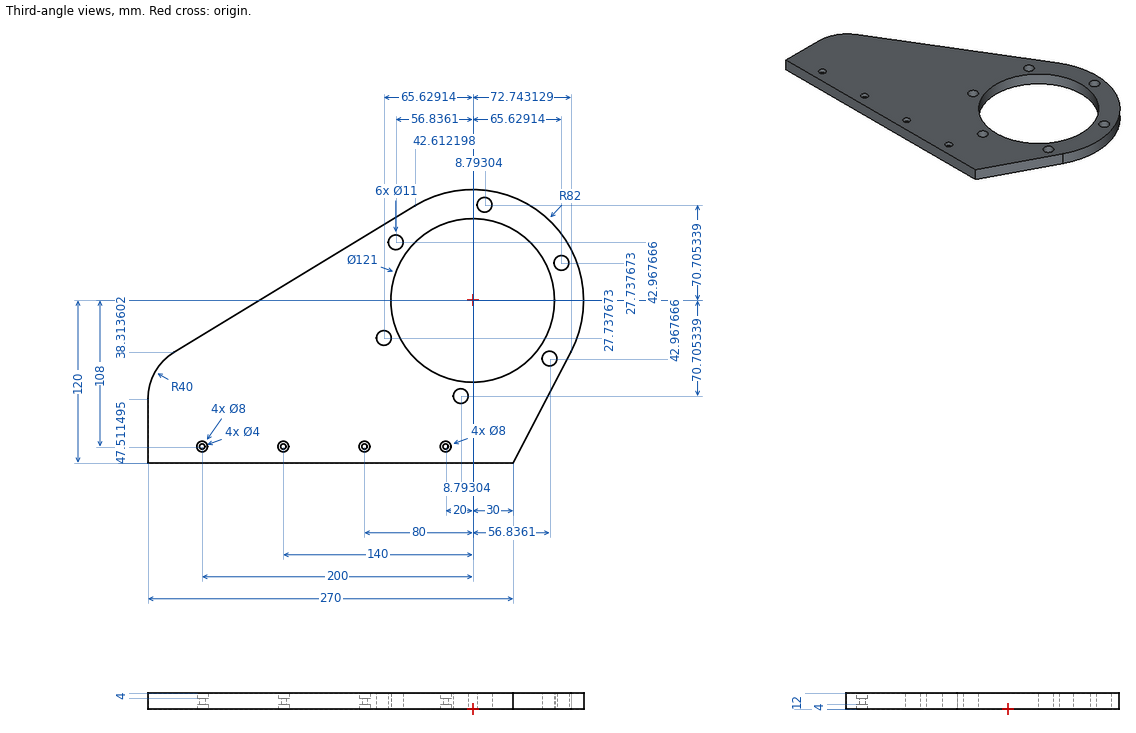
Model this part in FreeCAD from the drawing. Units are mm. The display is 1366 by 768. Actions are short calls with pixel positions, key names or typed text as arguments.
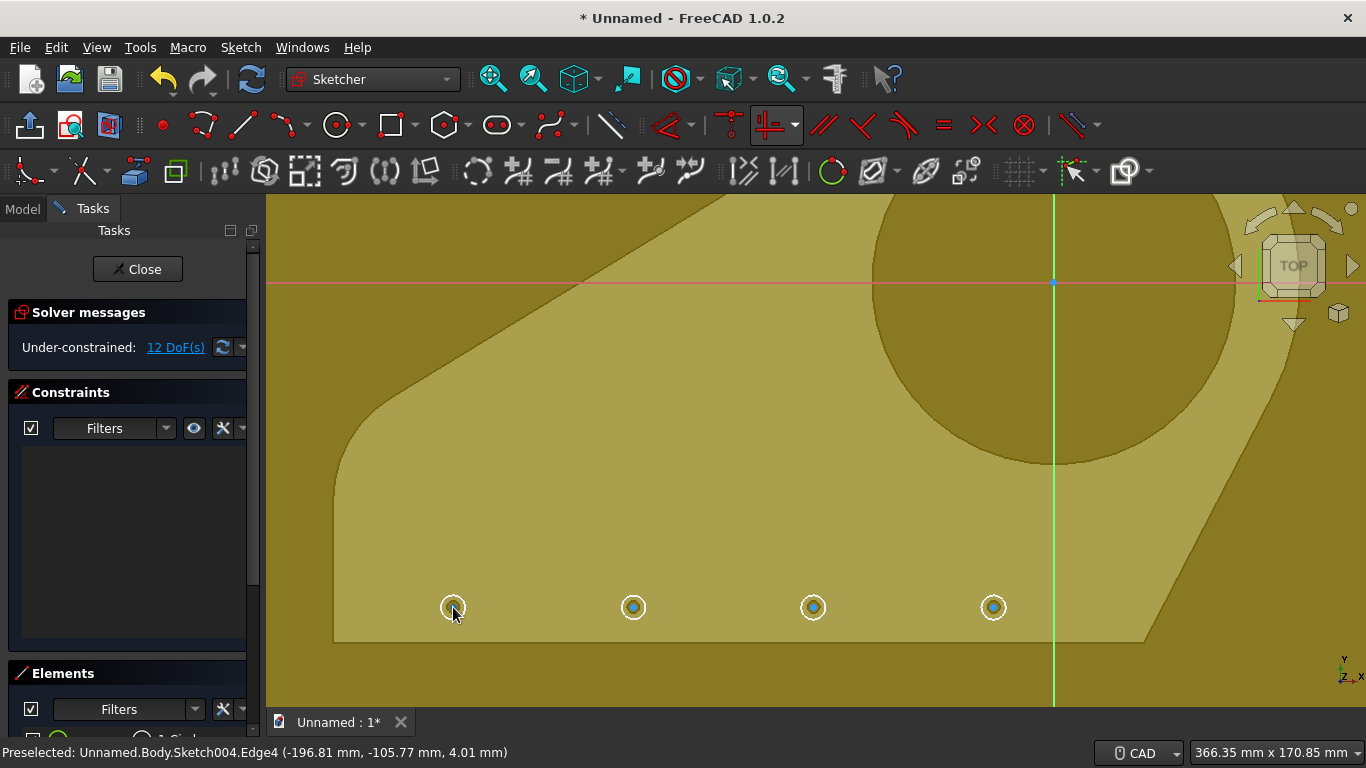
click(1002, 599)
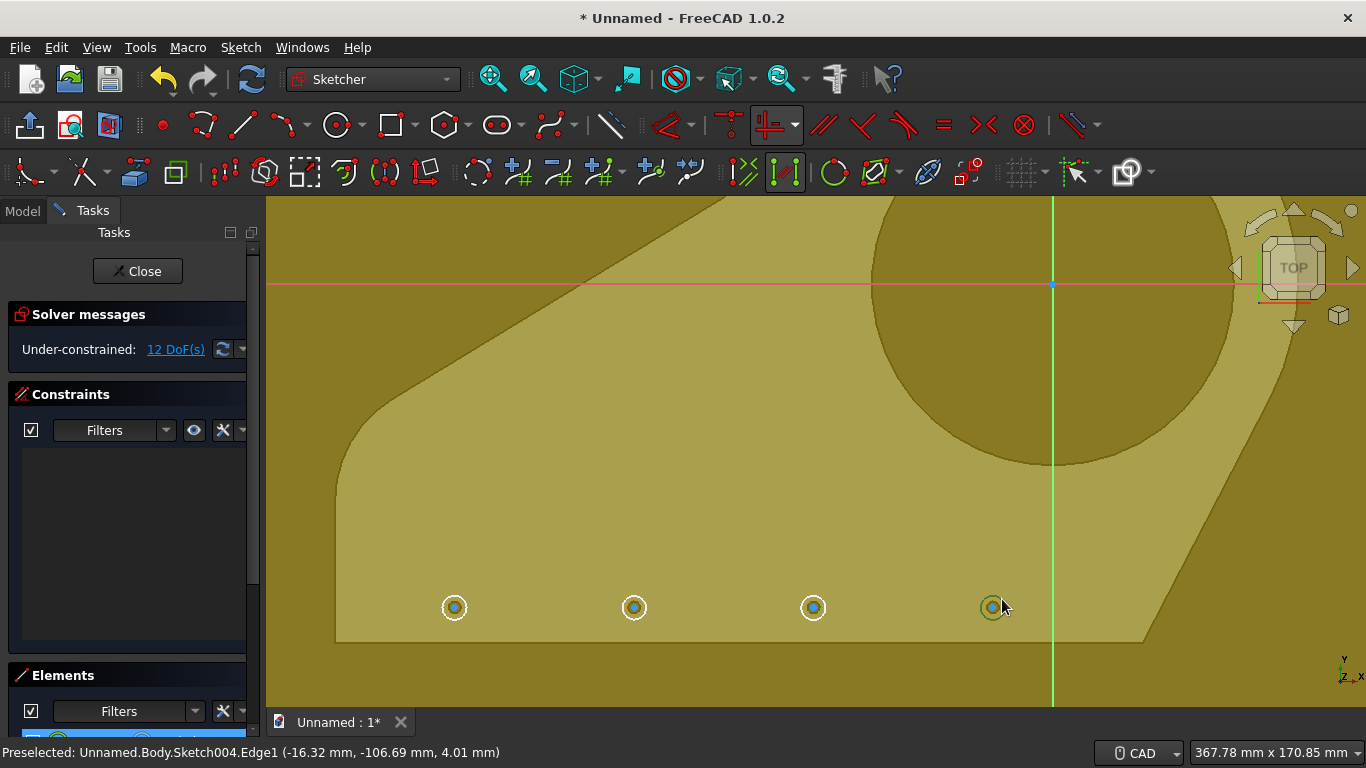
click(822, 599)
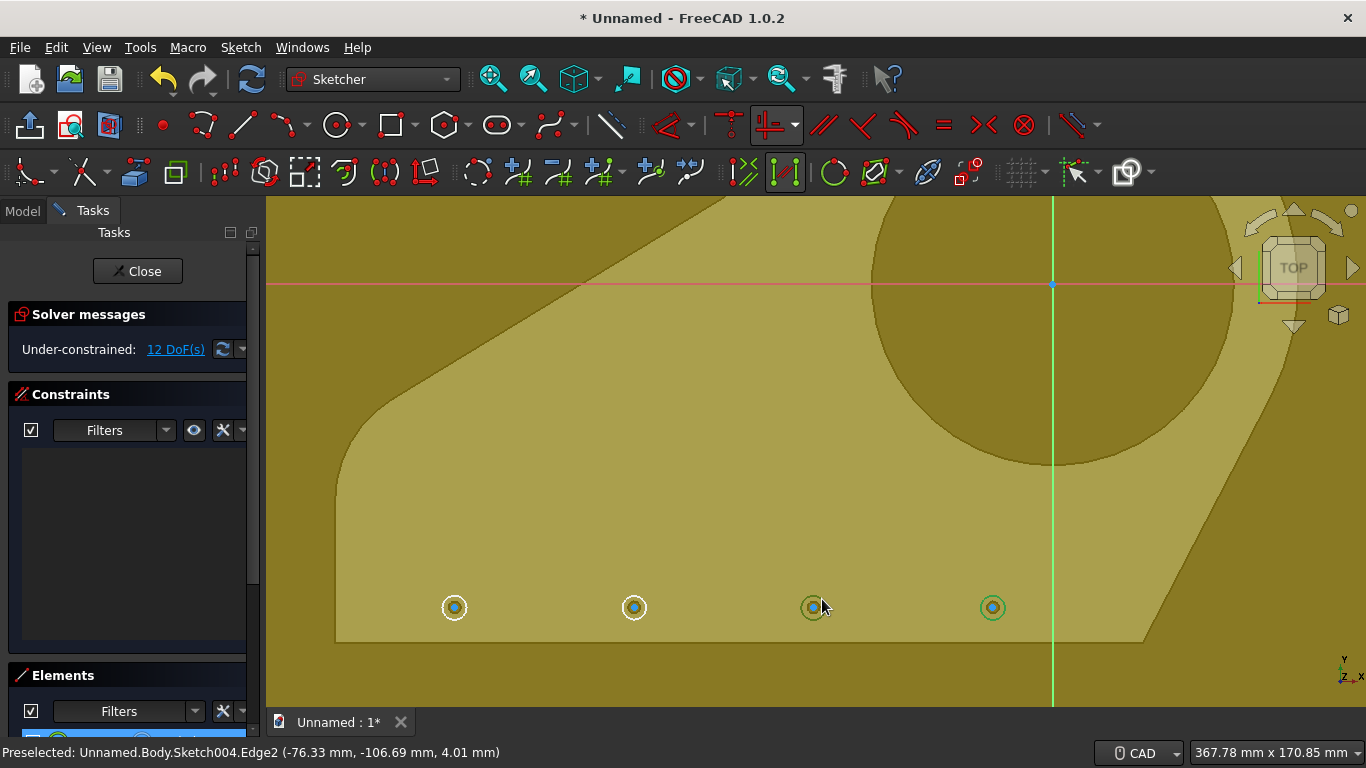
click(643, 600)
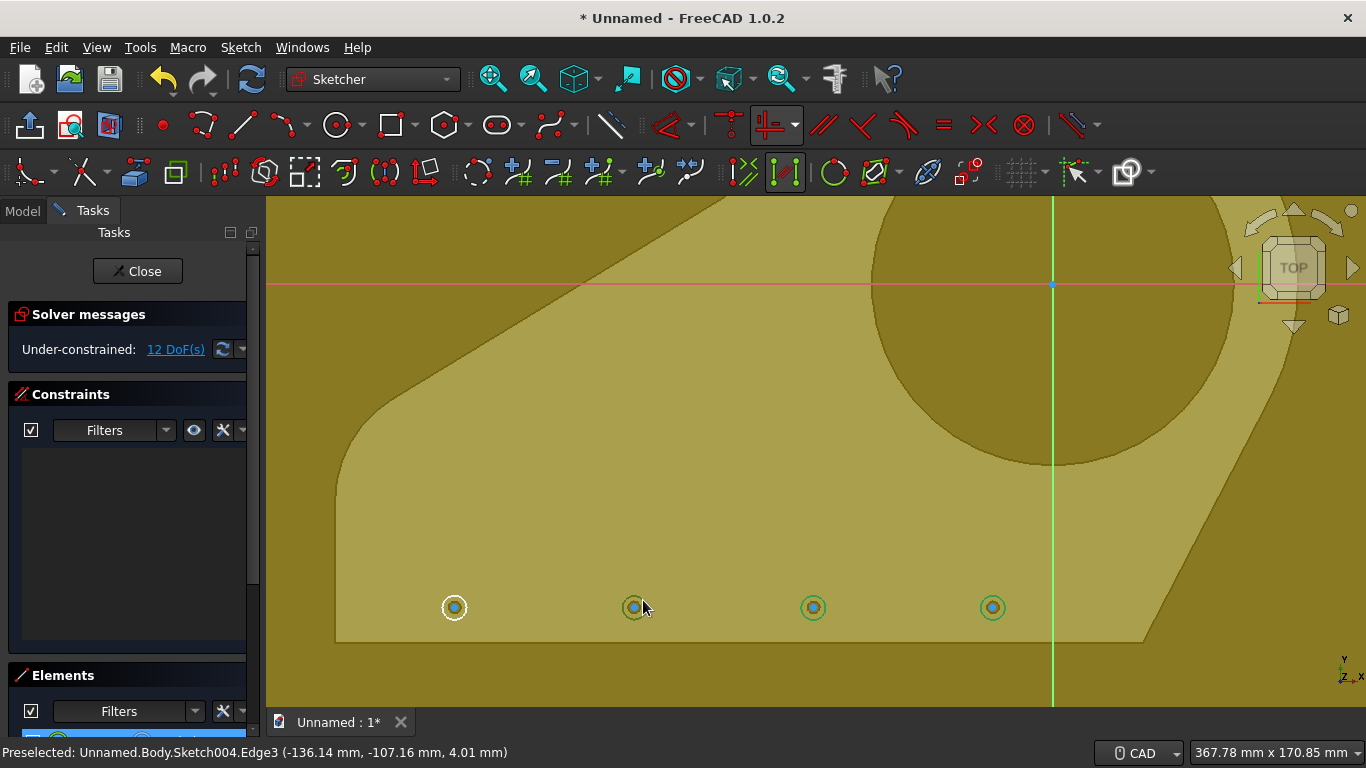
click(463, 599)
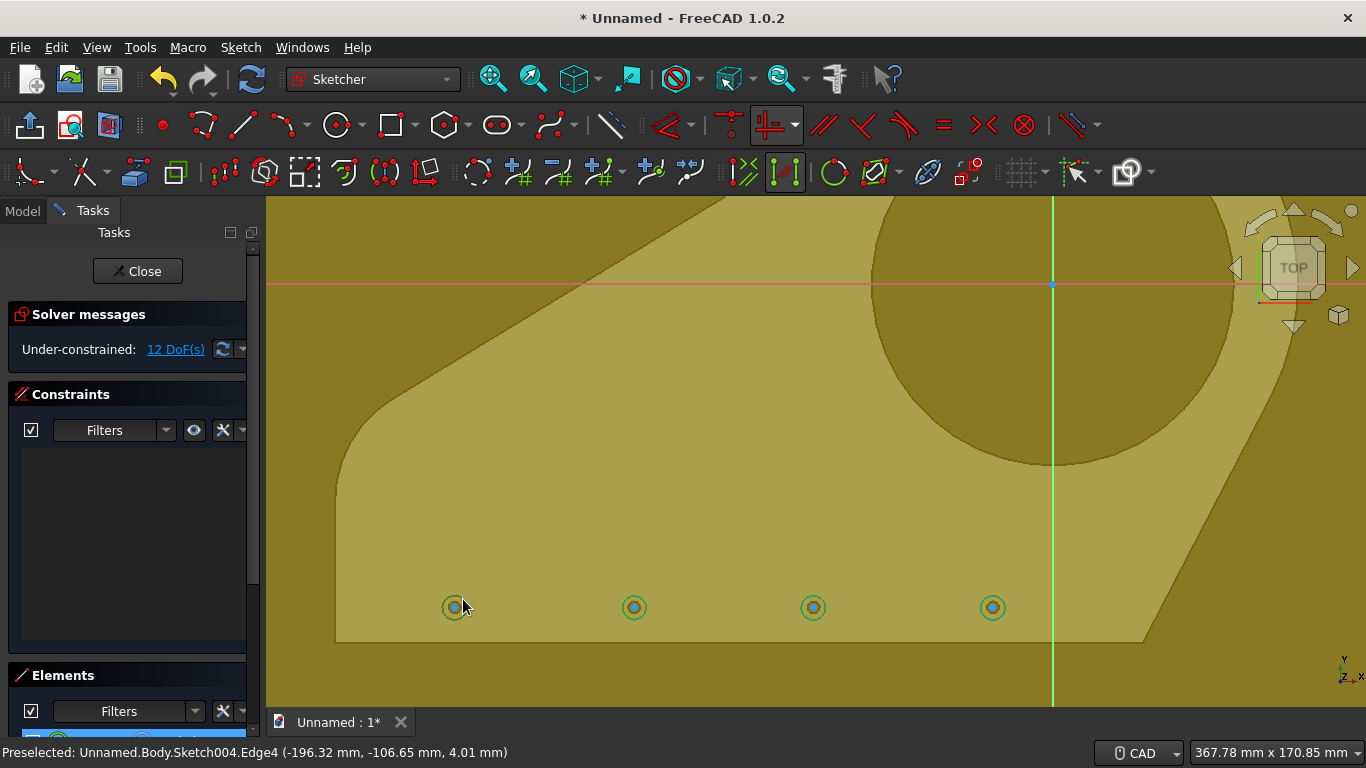
click(944, 126)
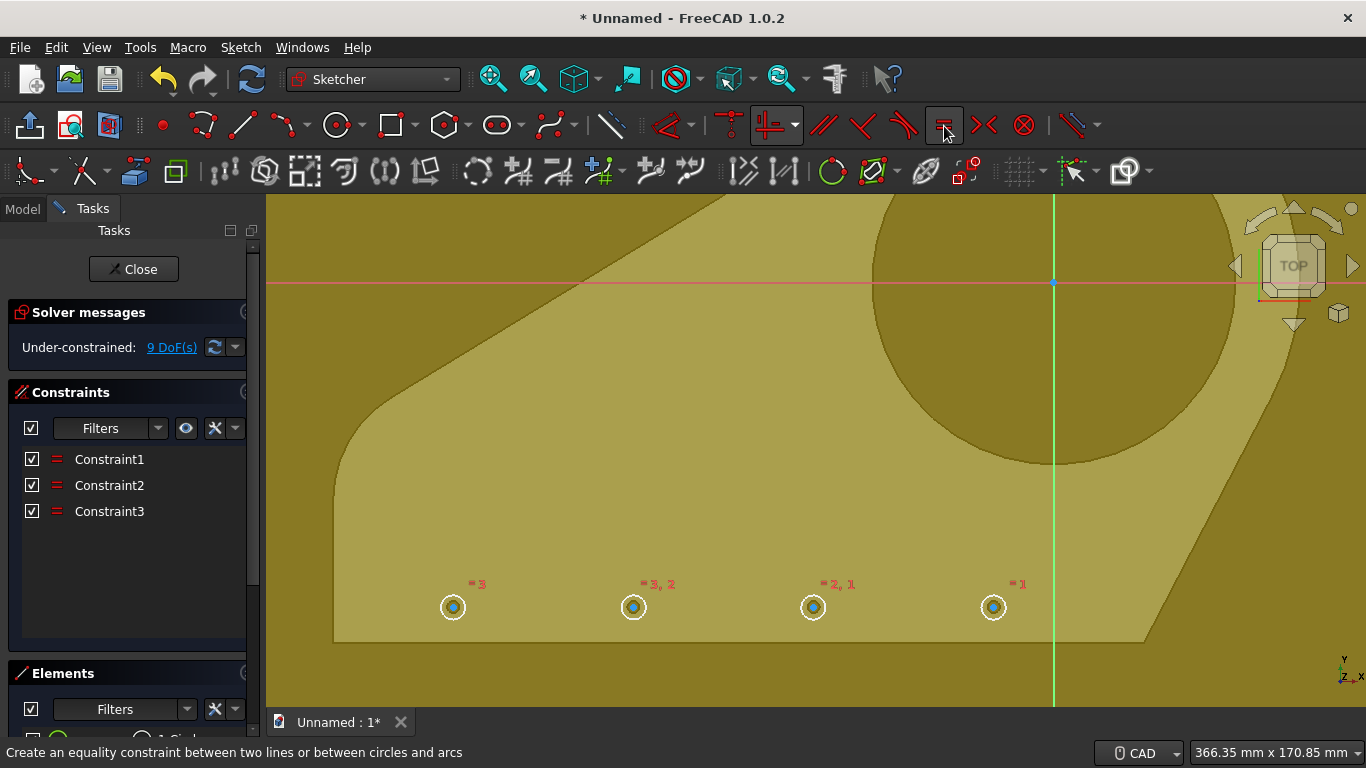
click(994, 608)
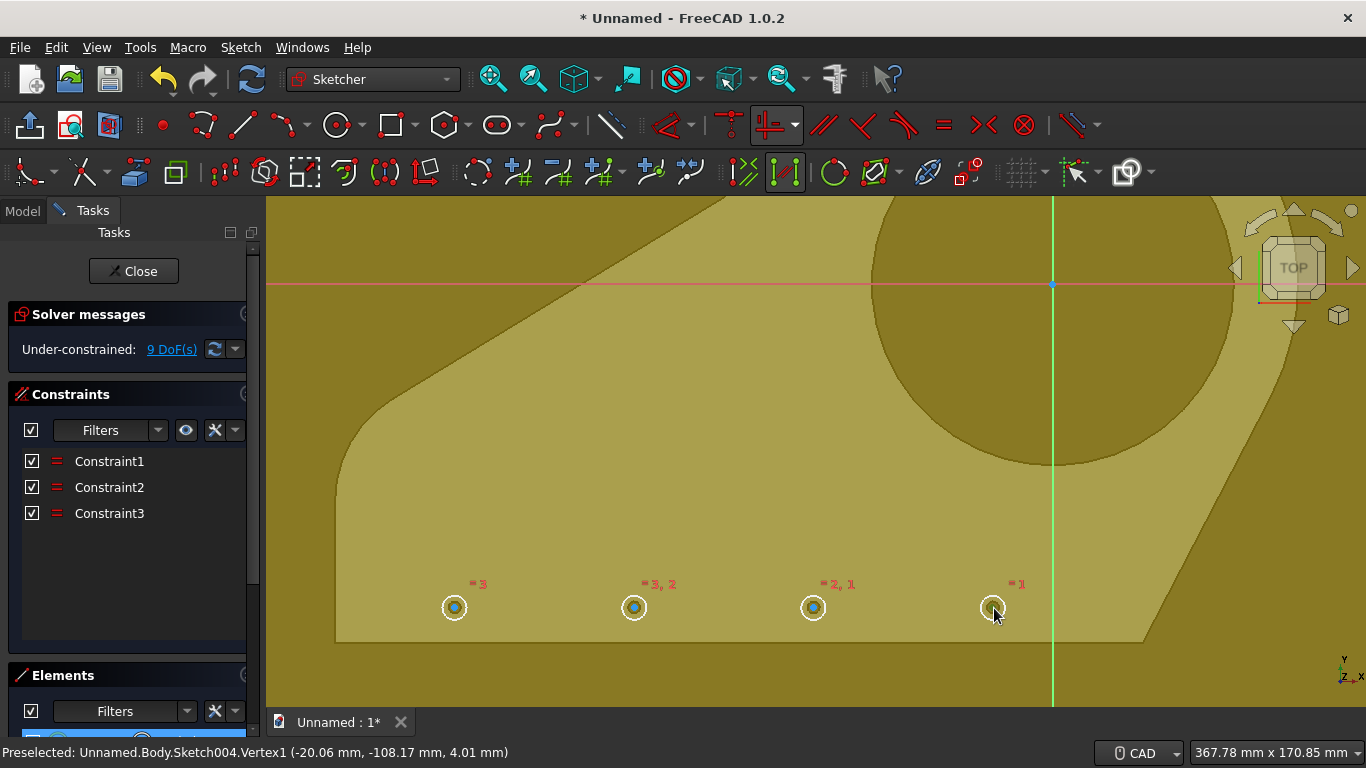
click(813, 608)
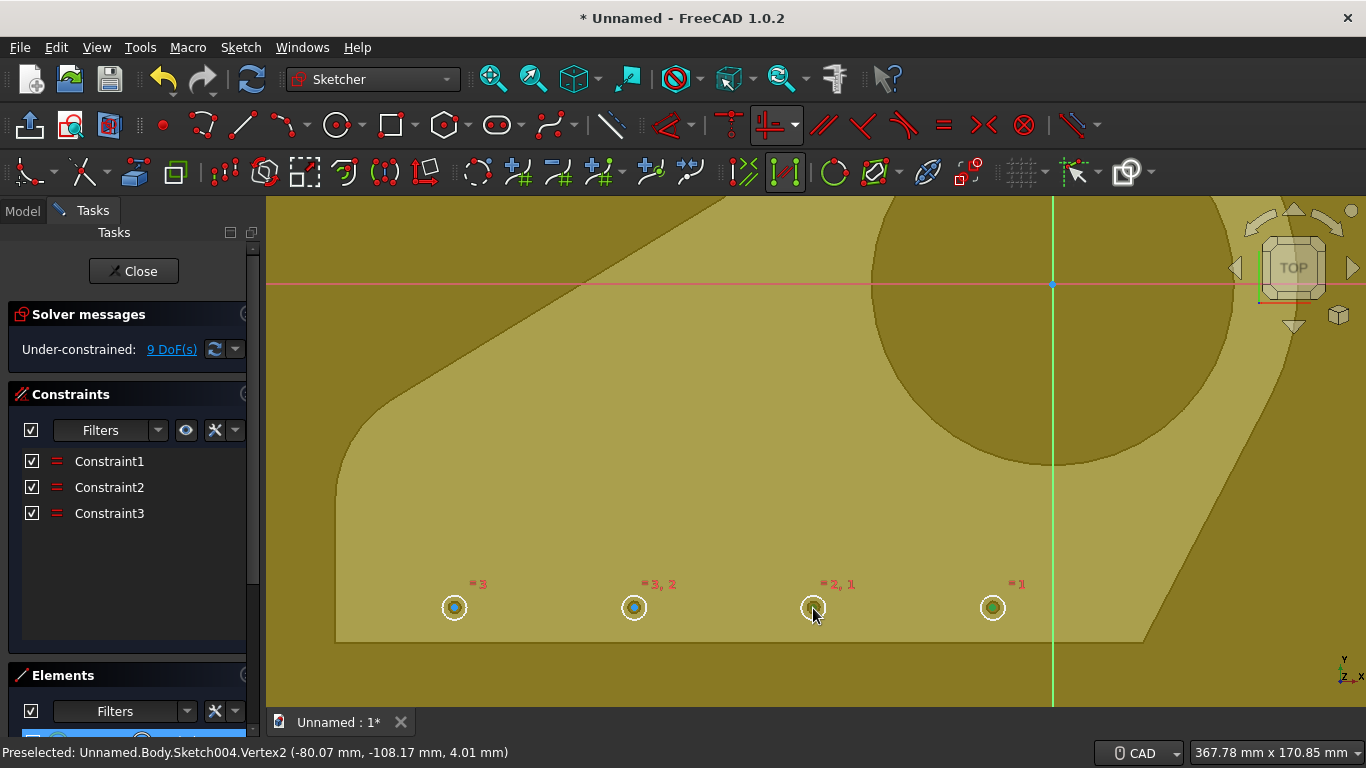
key(h)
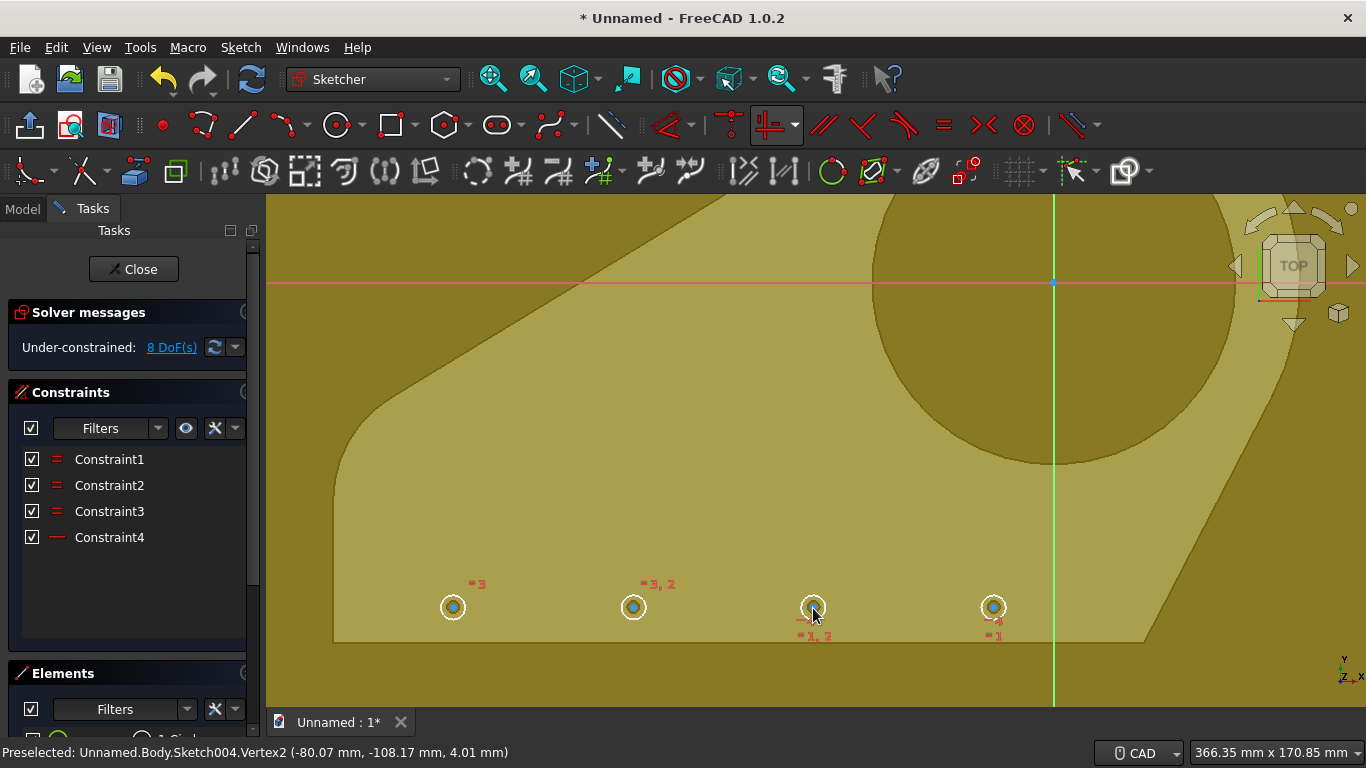
click(813, 608)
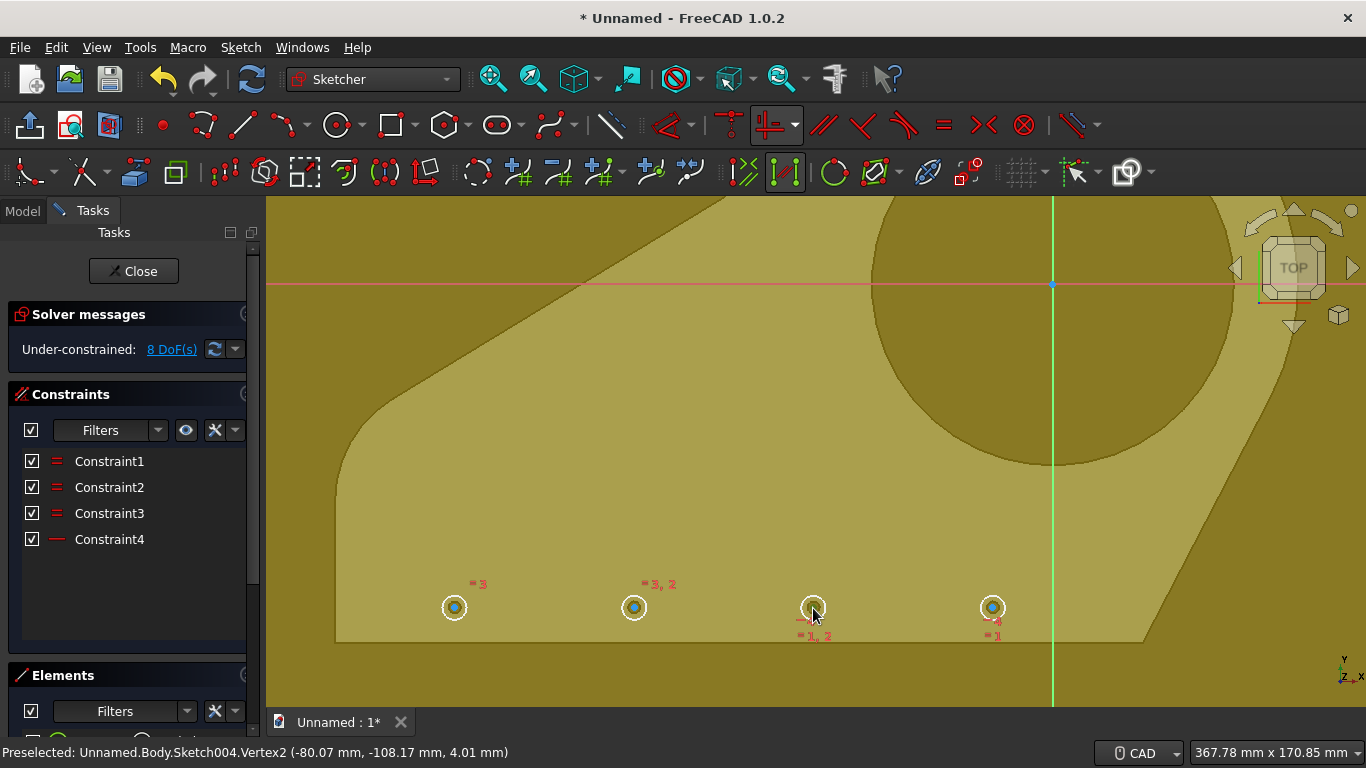
click(634, 608)